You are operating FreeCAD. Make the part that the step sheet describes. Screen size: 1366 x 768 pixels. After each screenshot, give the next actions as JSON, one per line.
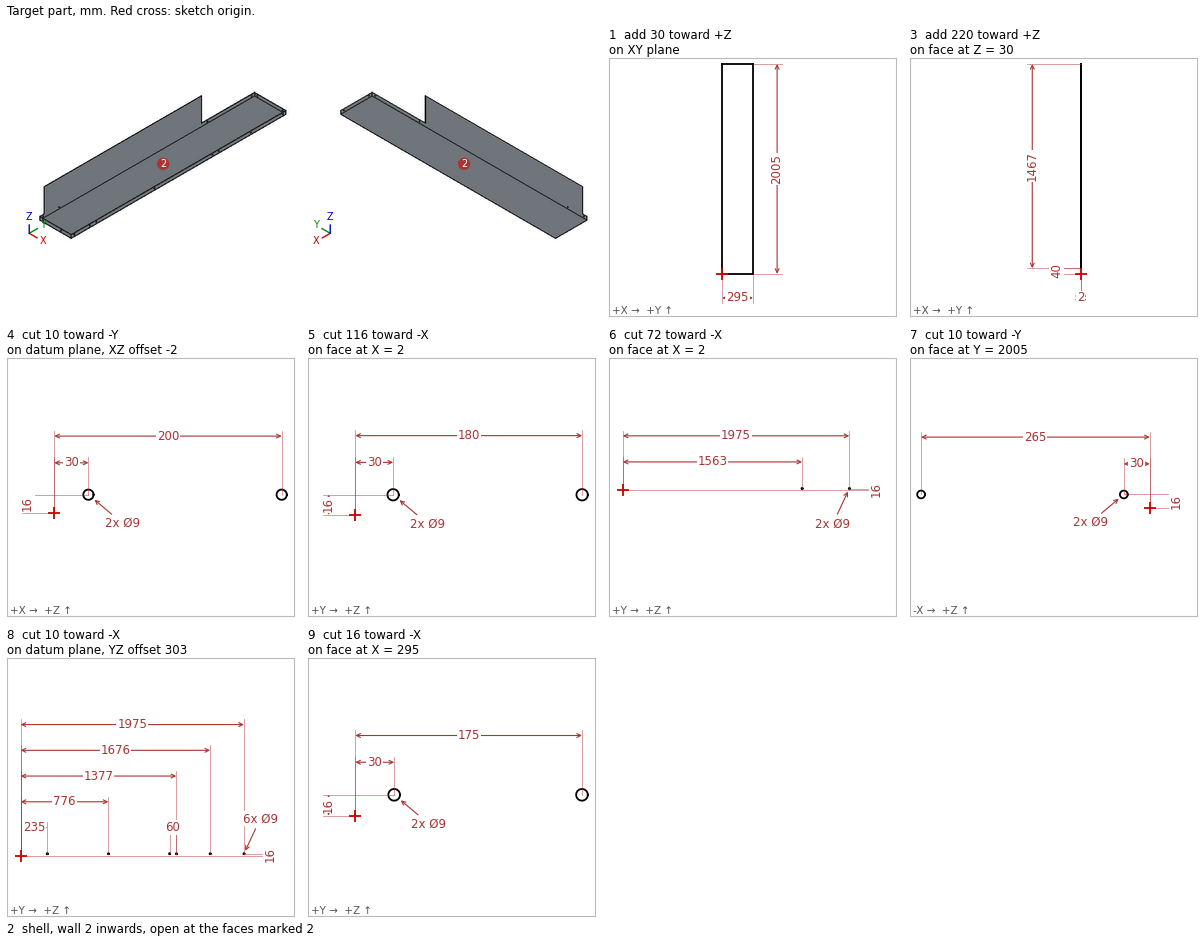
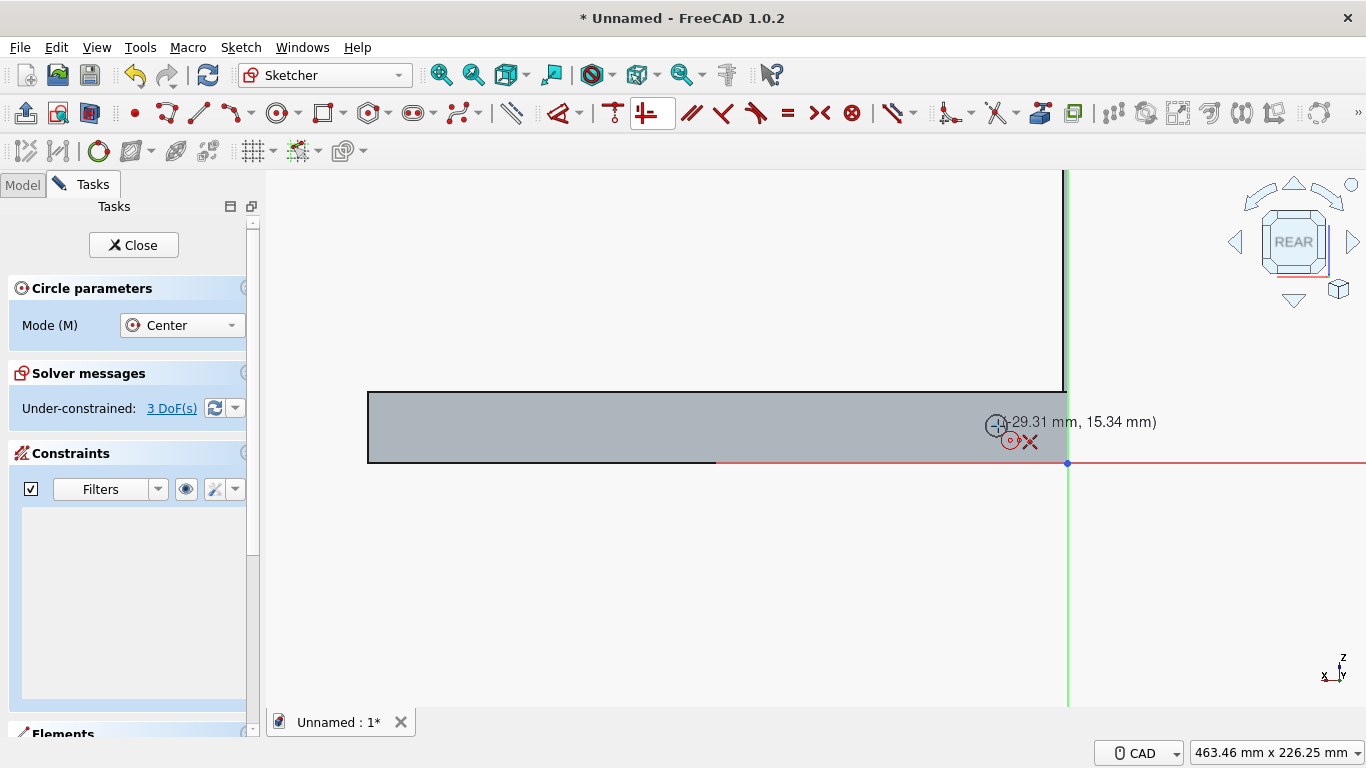
{"action": "scroll", "coordinate": [439, 425], "scroll_direction": "up", "scroll_amount": 4}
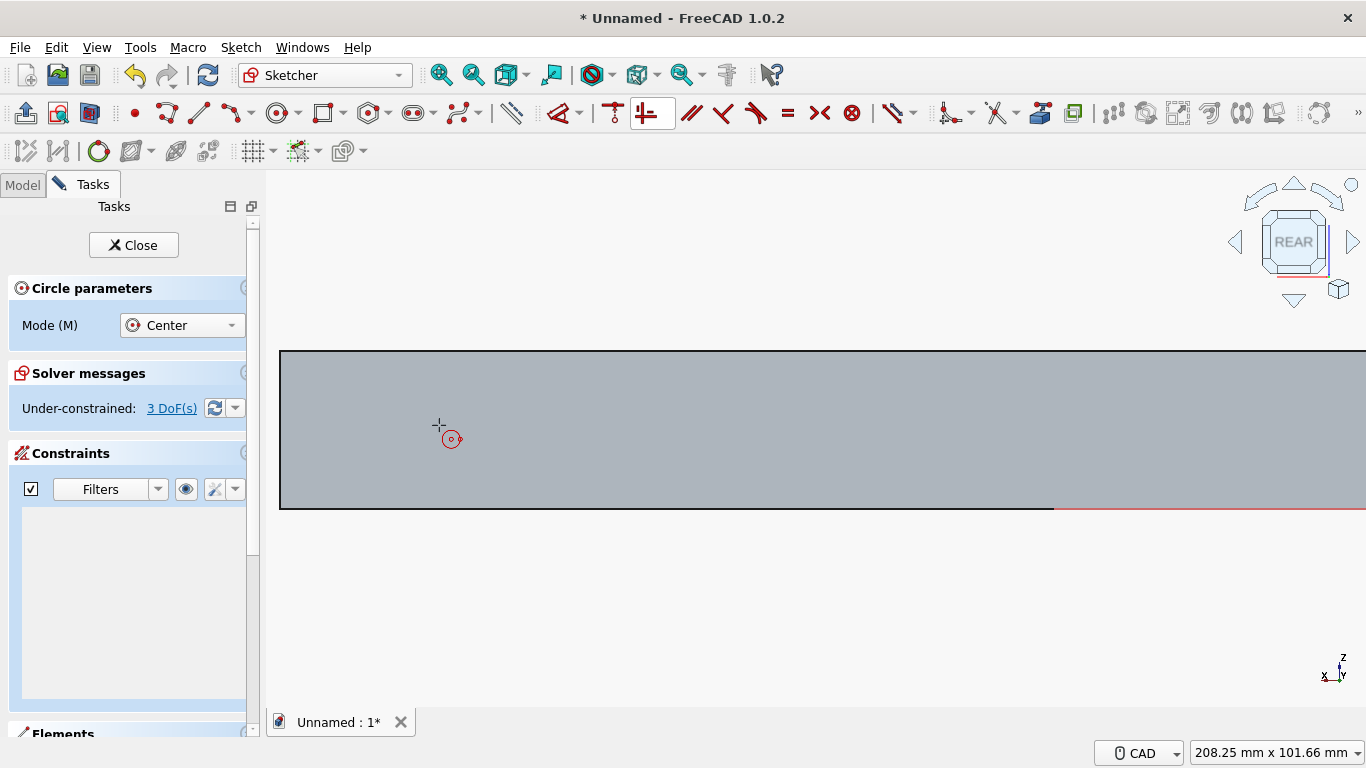
{"action": "left_click", "coordinate": [439, 425]}
{"action": "left_click", "coordinate": [456, 408]}
{"action": "key", "text": "Escape"}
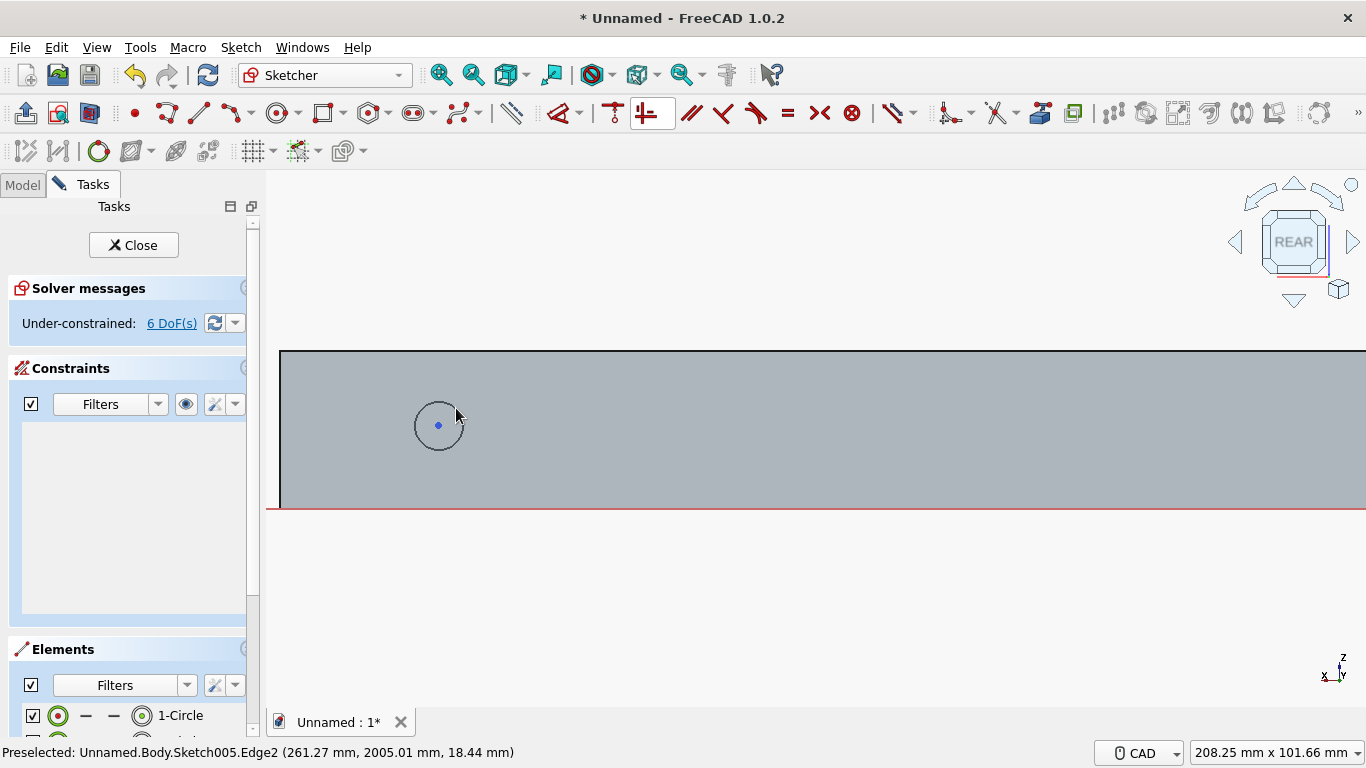
{"action": "scroll", "coordinate": [438, 425], "scroll_direction": "down", "scroll_amount": 4}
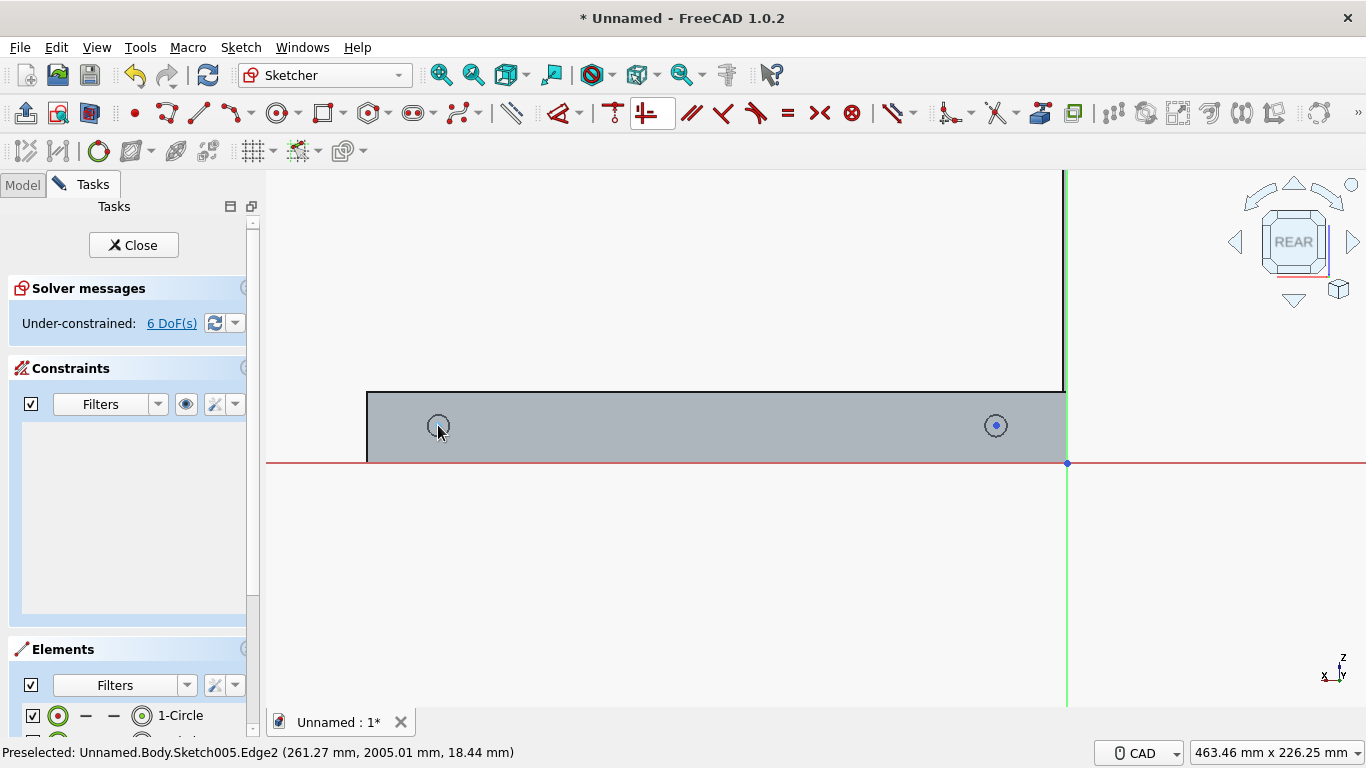
{"action": "scroll", "coordinate": [1004, 418], "scroll_direction": "up", "scroll_amount": 2}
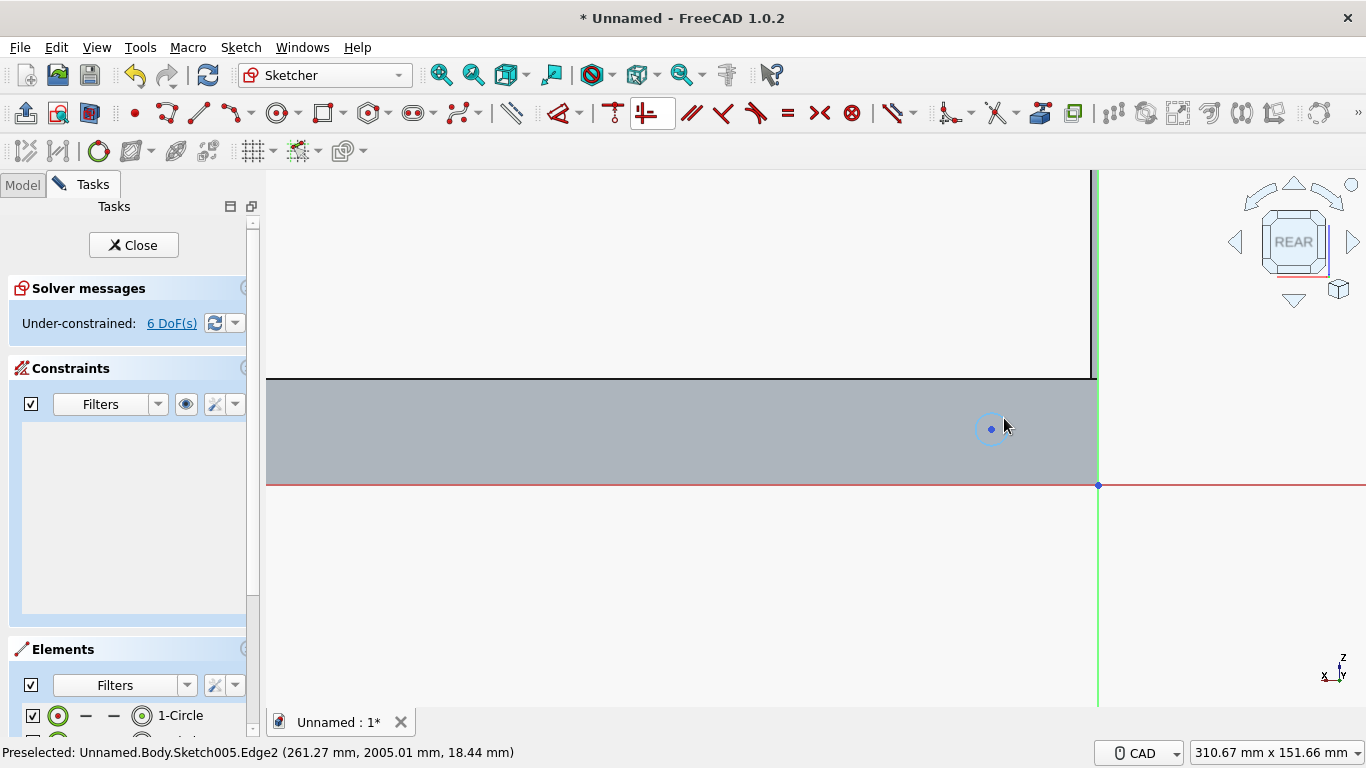
{"action": "left_click", "coordinate": [1003, 418]}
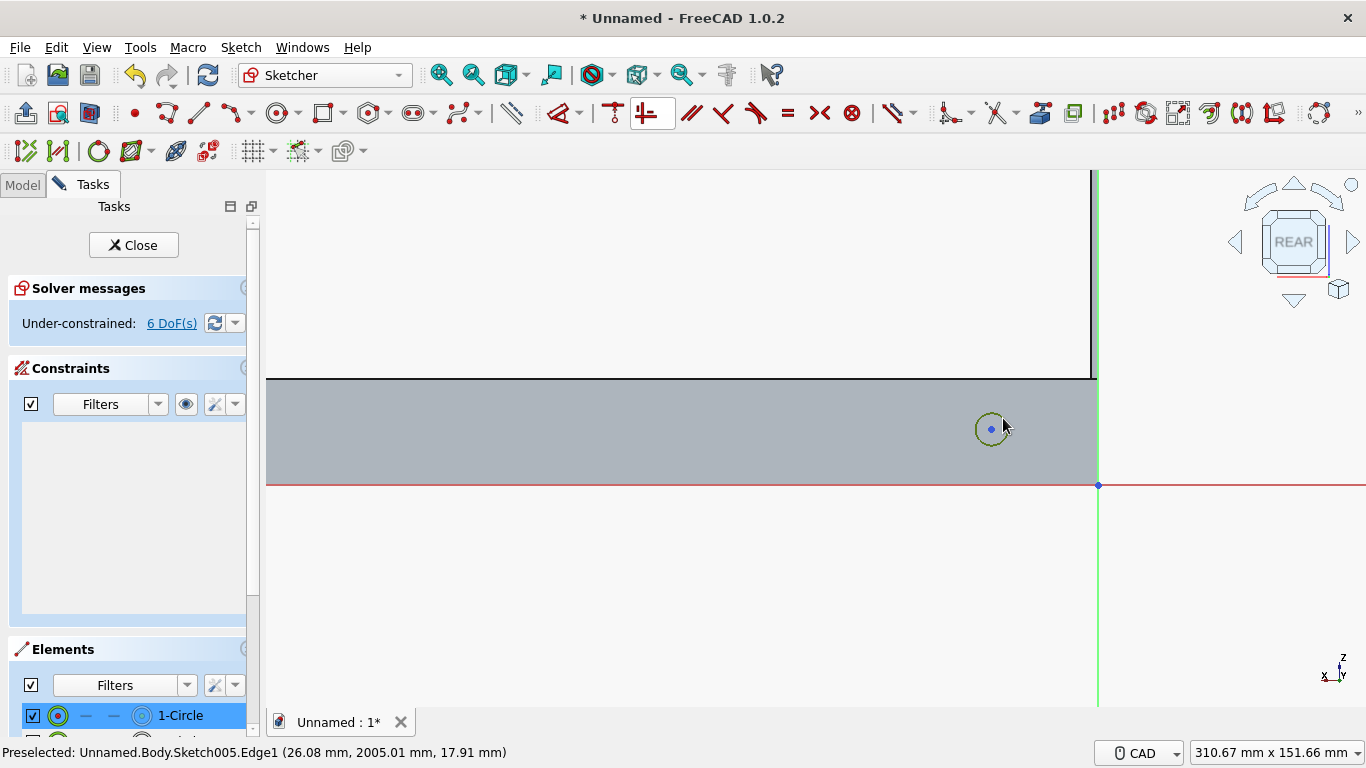
{"action": "scroll", "coordinate": [1004, 418], "scroll_direction": "down", "scroll_amount": 2}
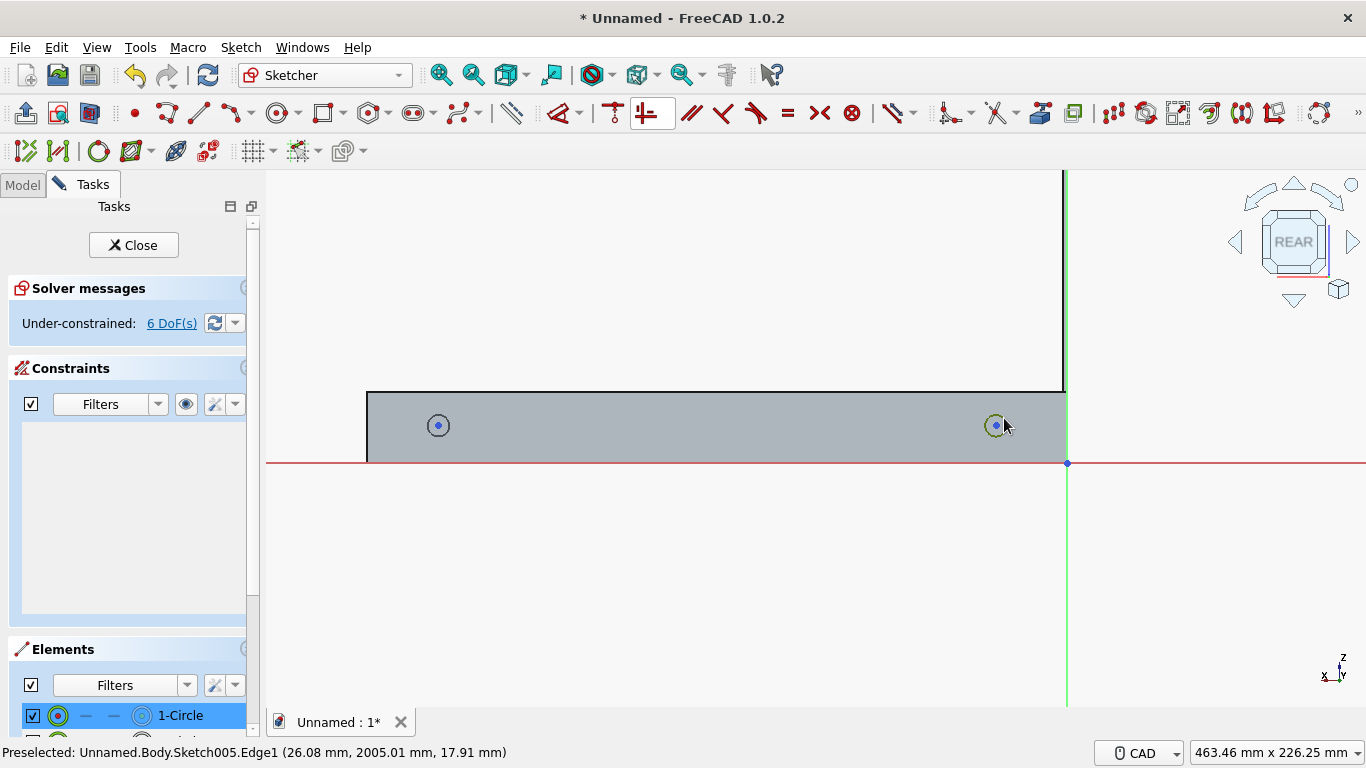
{"action": "scroll", "coordinate": [446, 418], "scroll_direction": "up", "scroll_amount": 2}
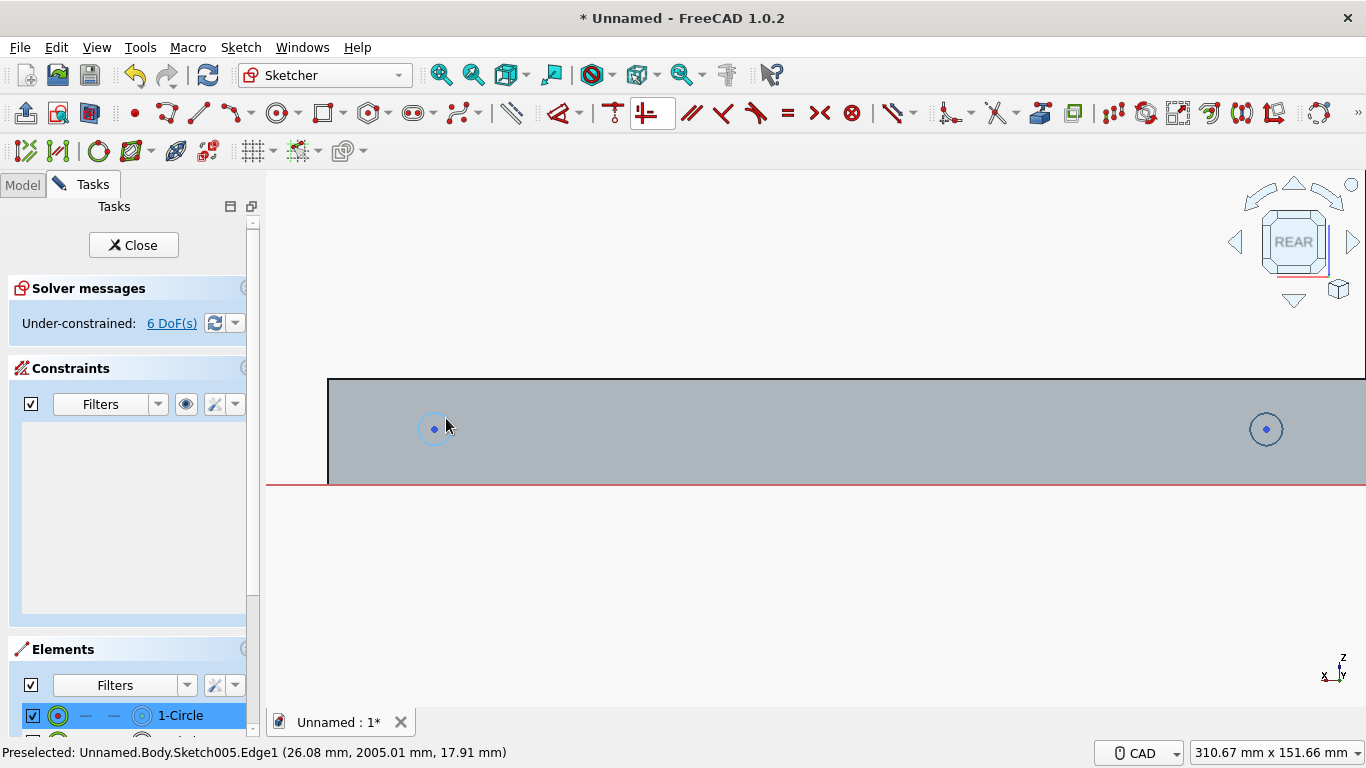
{"action": "left_click", "coordinate": [446, 418]}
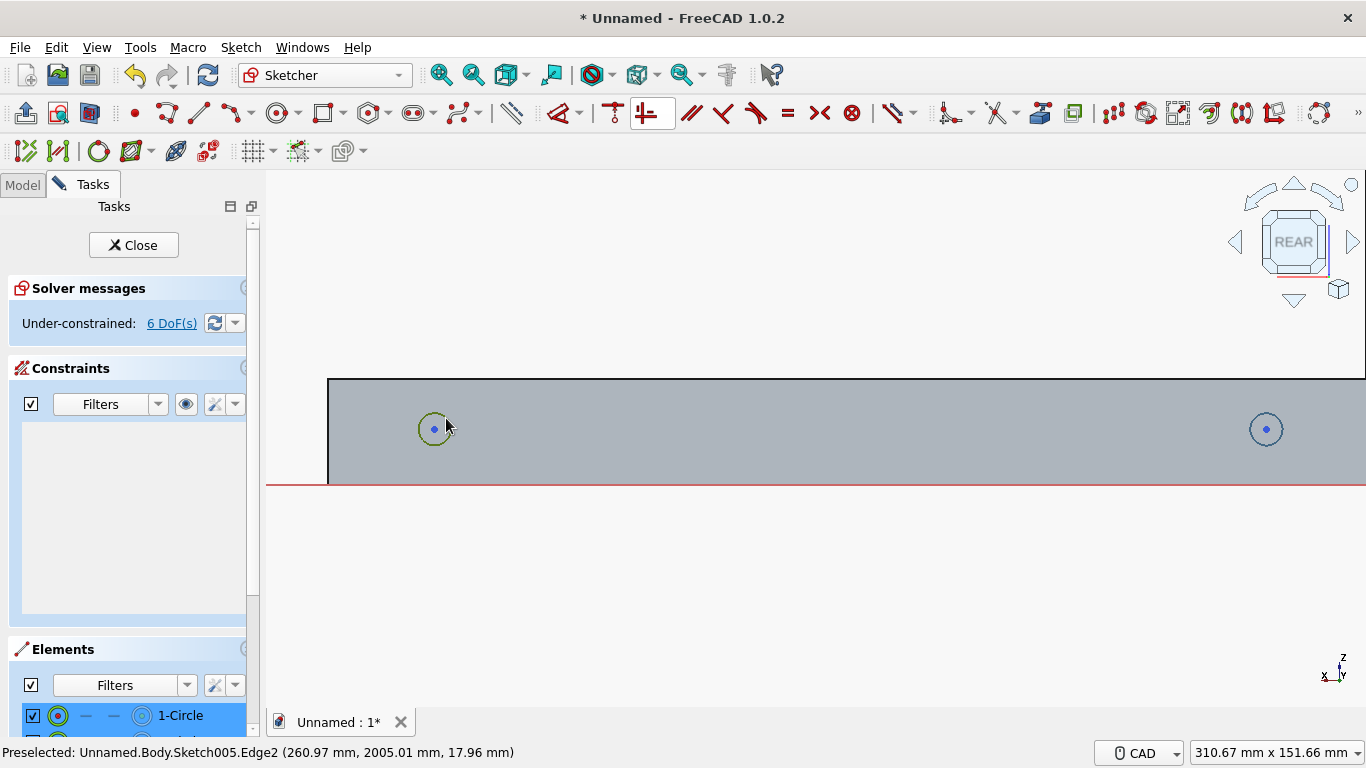
{"action": "key", "text": "e"}